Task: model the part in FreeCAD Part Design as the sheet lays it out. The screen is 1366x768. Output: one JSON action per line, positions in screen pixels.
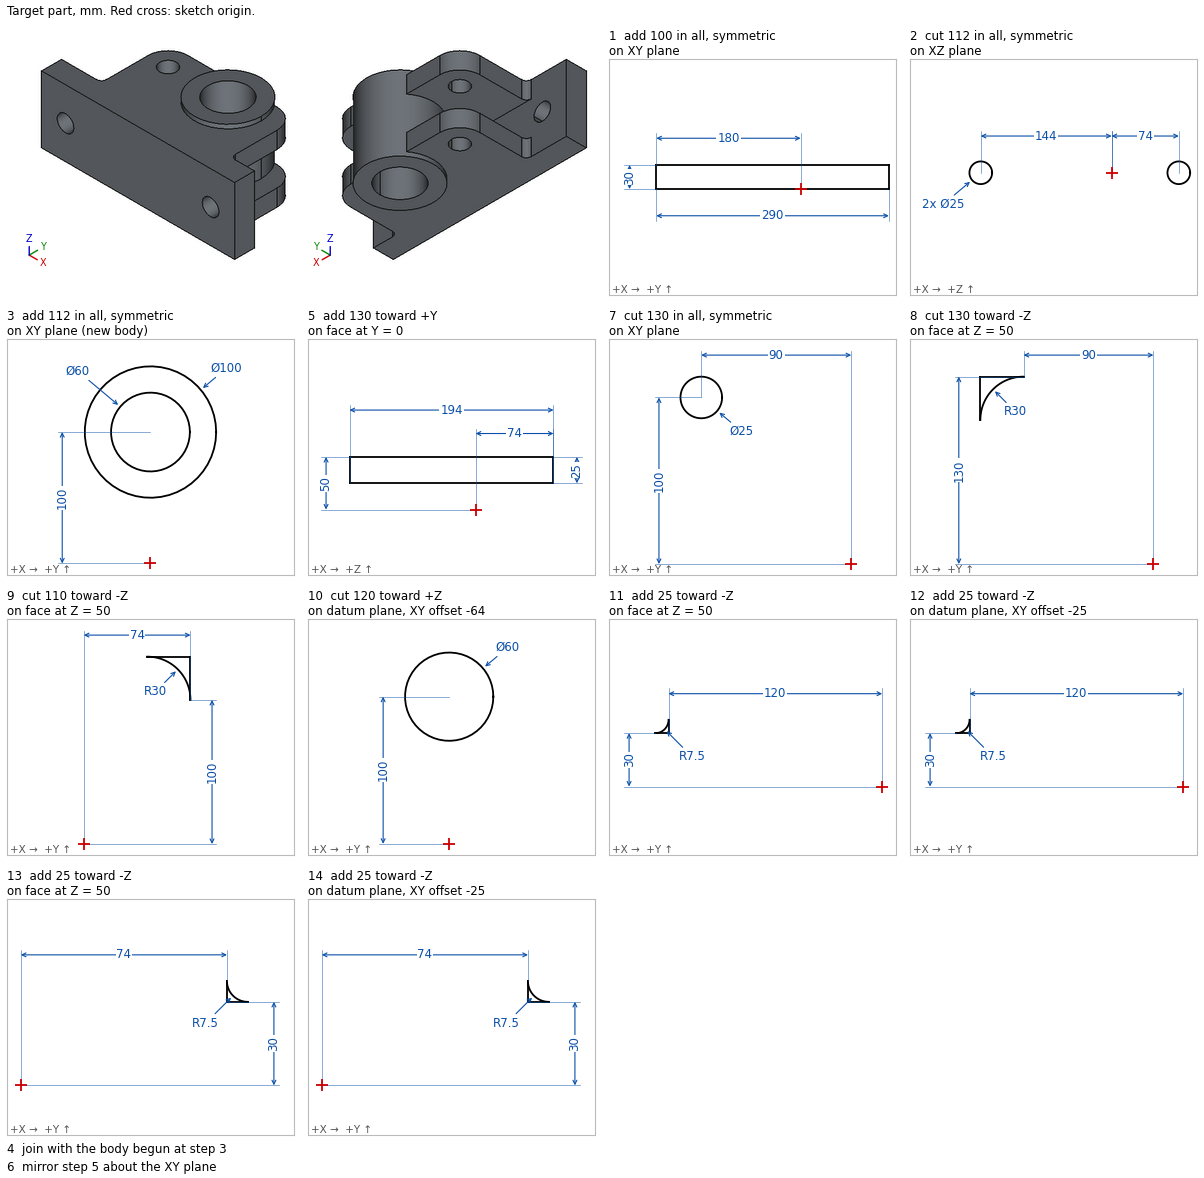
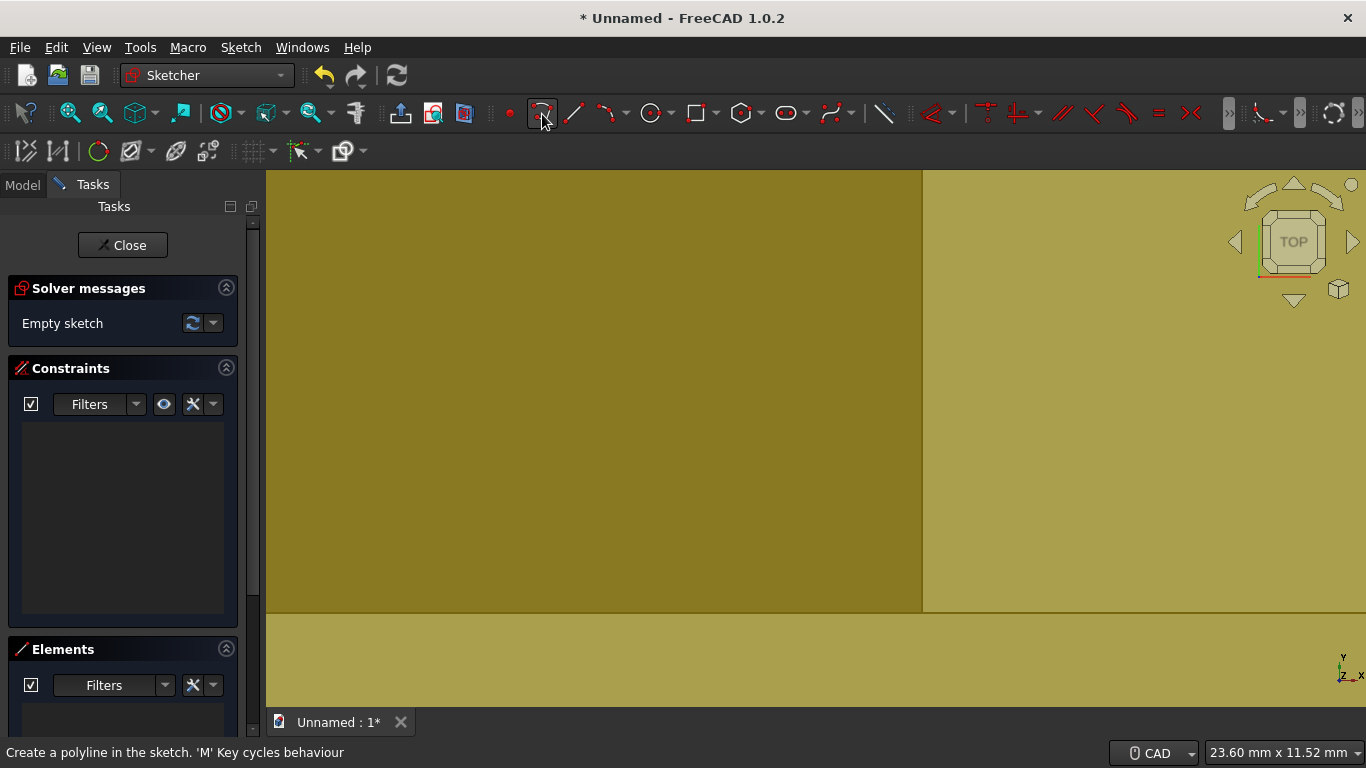
{"action": "left_click", "coordinate": [572, 613]}
{"action": "left_click", "coordinate": [922, 613]}
{"action": "left_click", "coordinate": [922, 264]}
{"action": "right_click", "coordinate": [922, 264]}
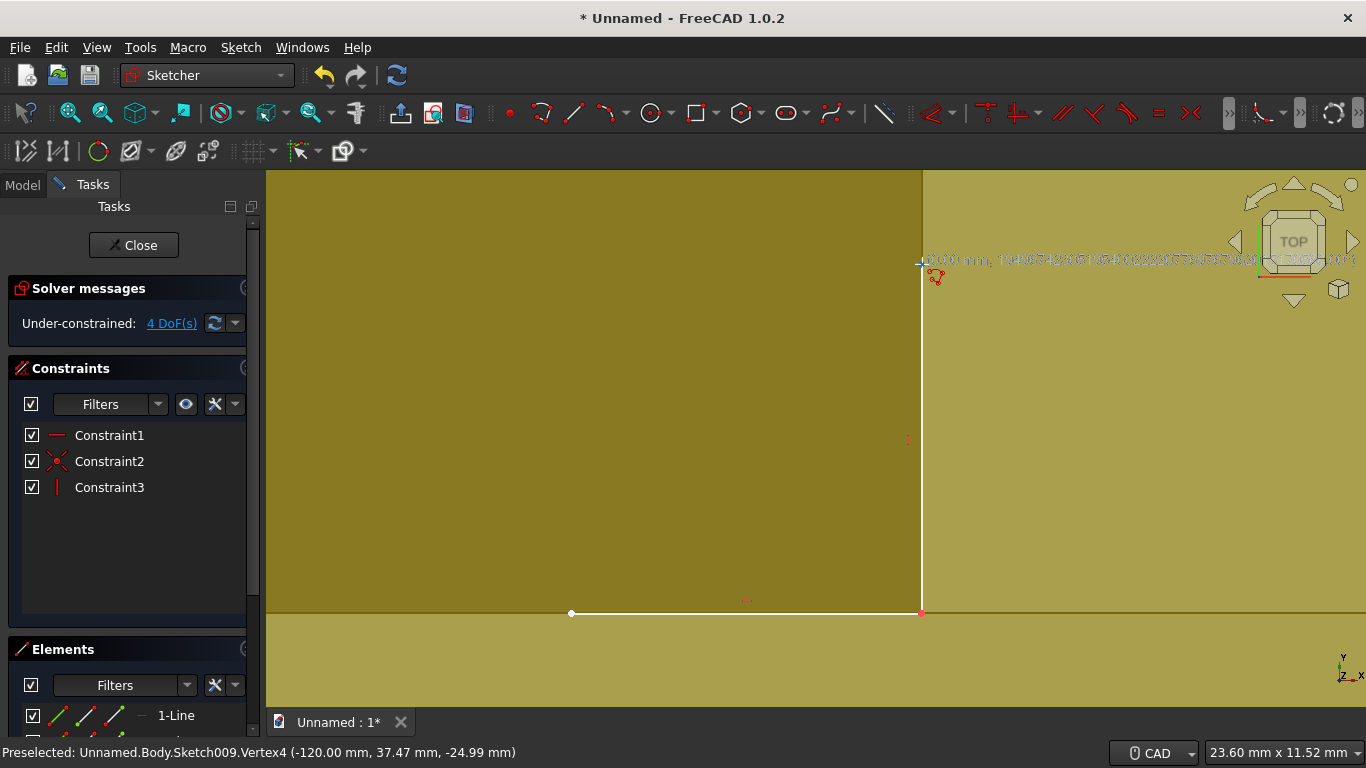
{"action": "left_click", "coordinate": [606, 114]}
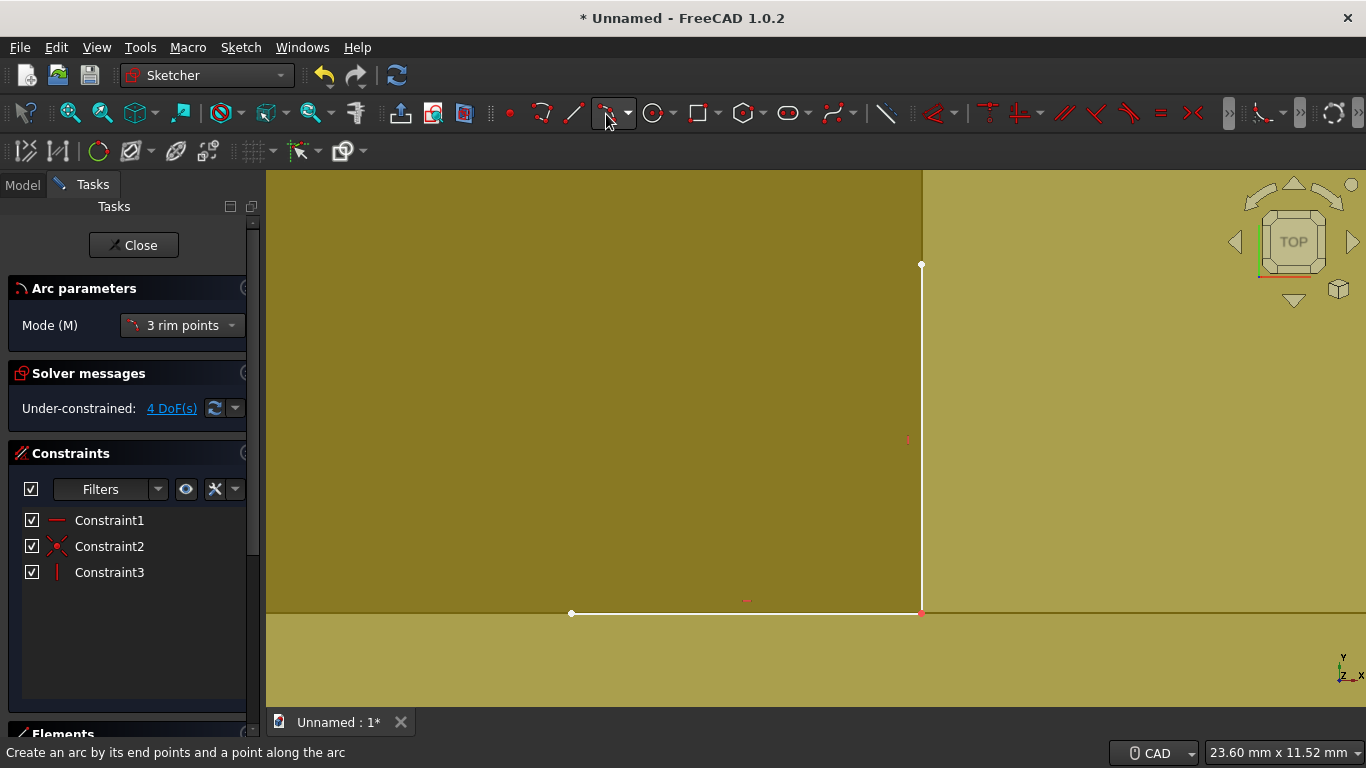
{"action": "left_click", "coordinate": [922, 265]}
{"action": "left_click", "coordinate": [572, 614]}
{"action": "left_click", "coordinate": [820, 511]}
{"action": "key", "text": "Escape"}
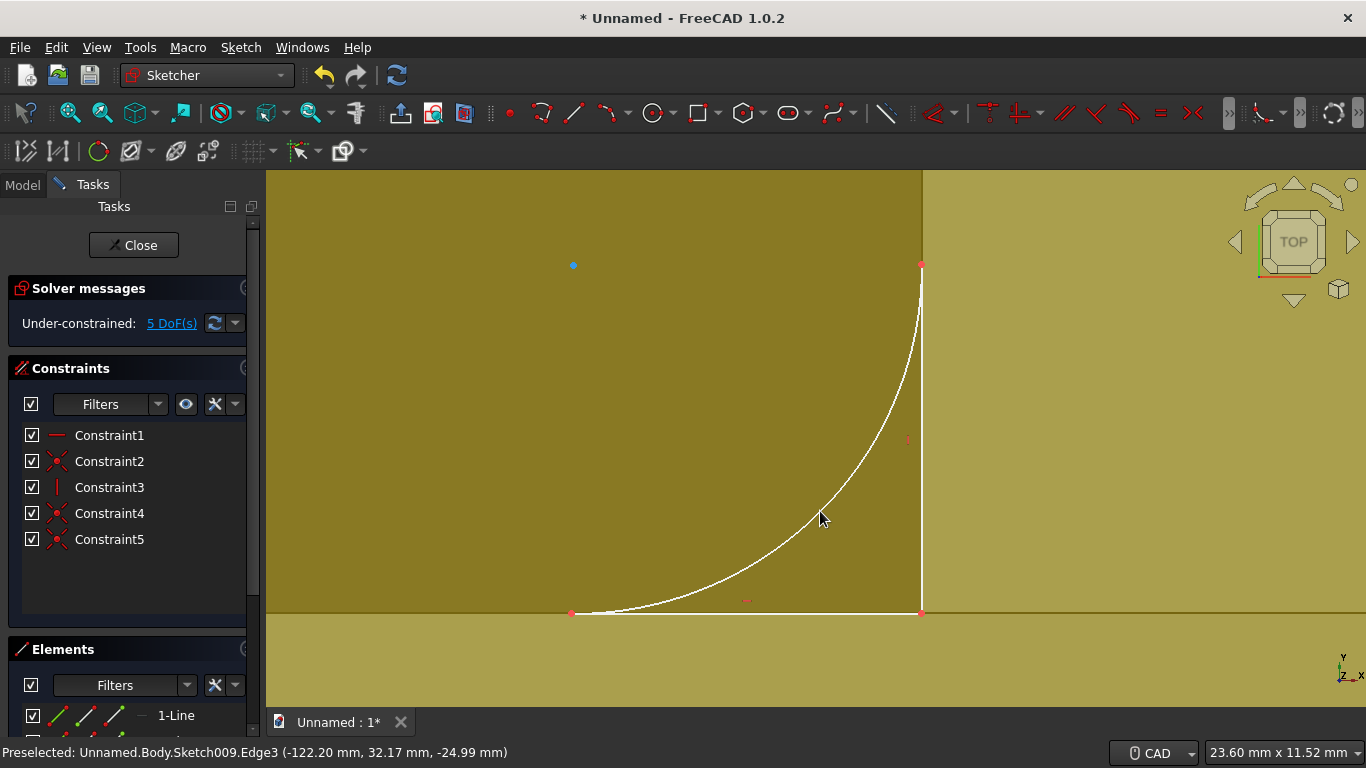
{"action": "left_click", "coordinate": [677, 614]}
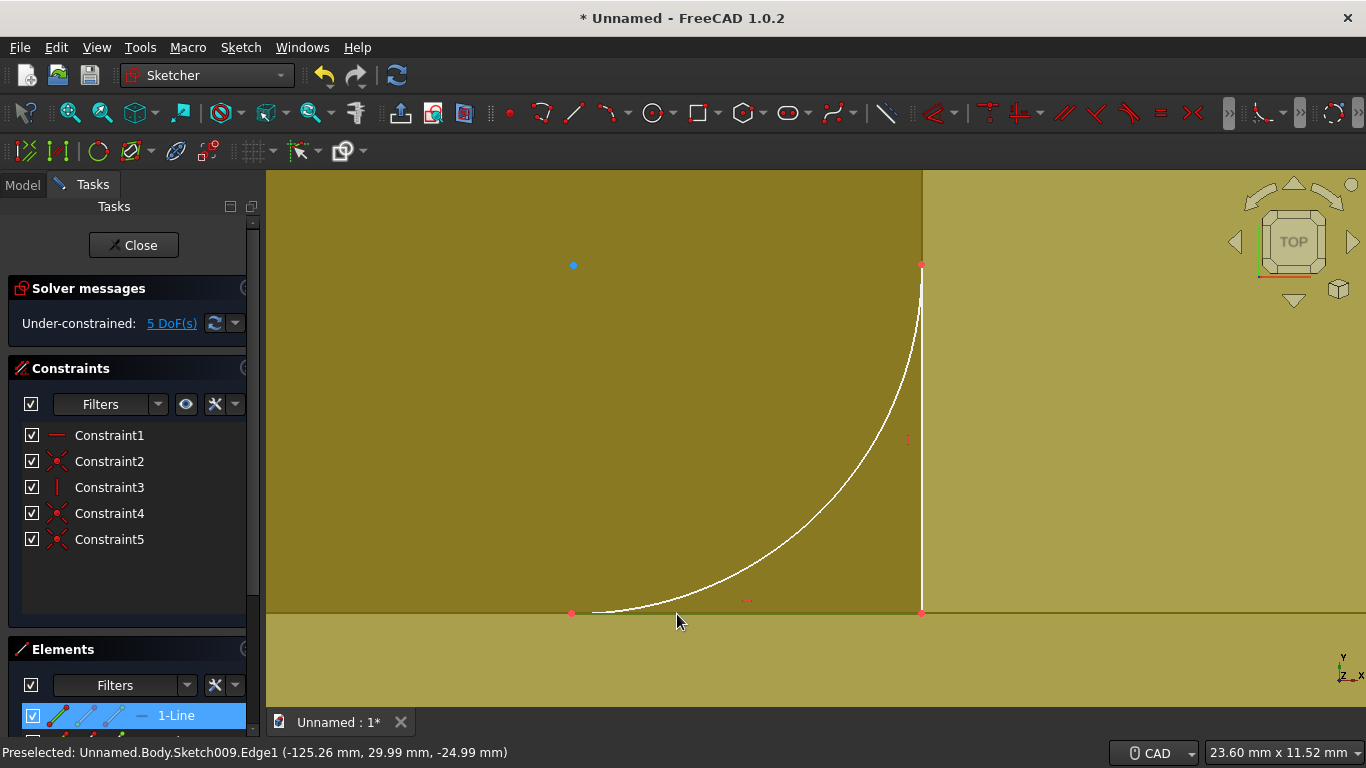
{"action": "left_click", "coordinate": [731, 576]}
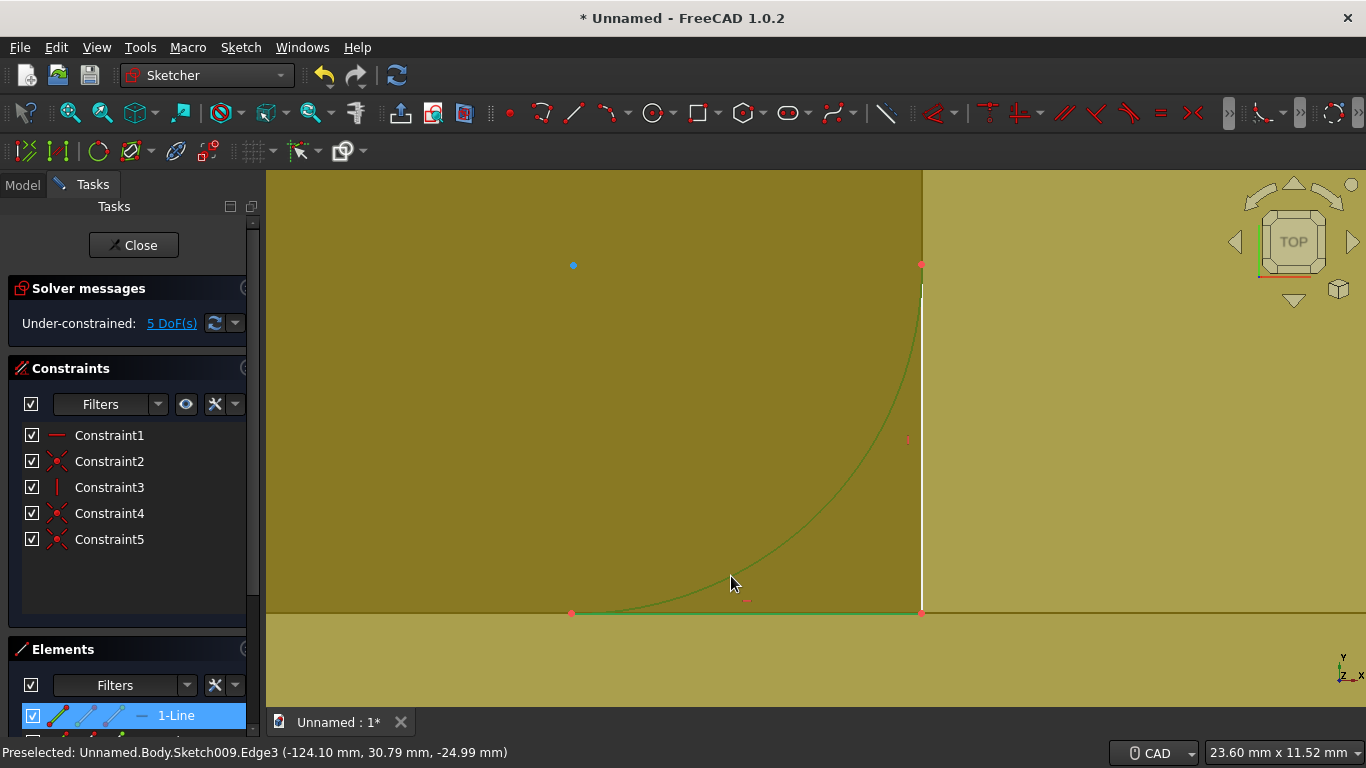
{"action": "left_click", "coordinate": [1130, 114]}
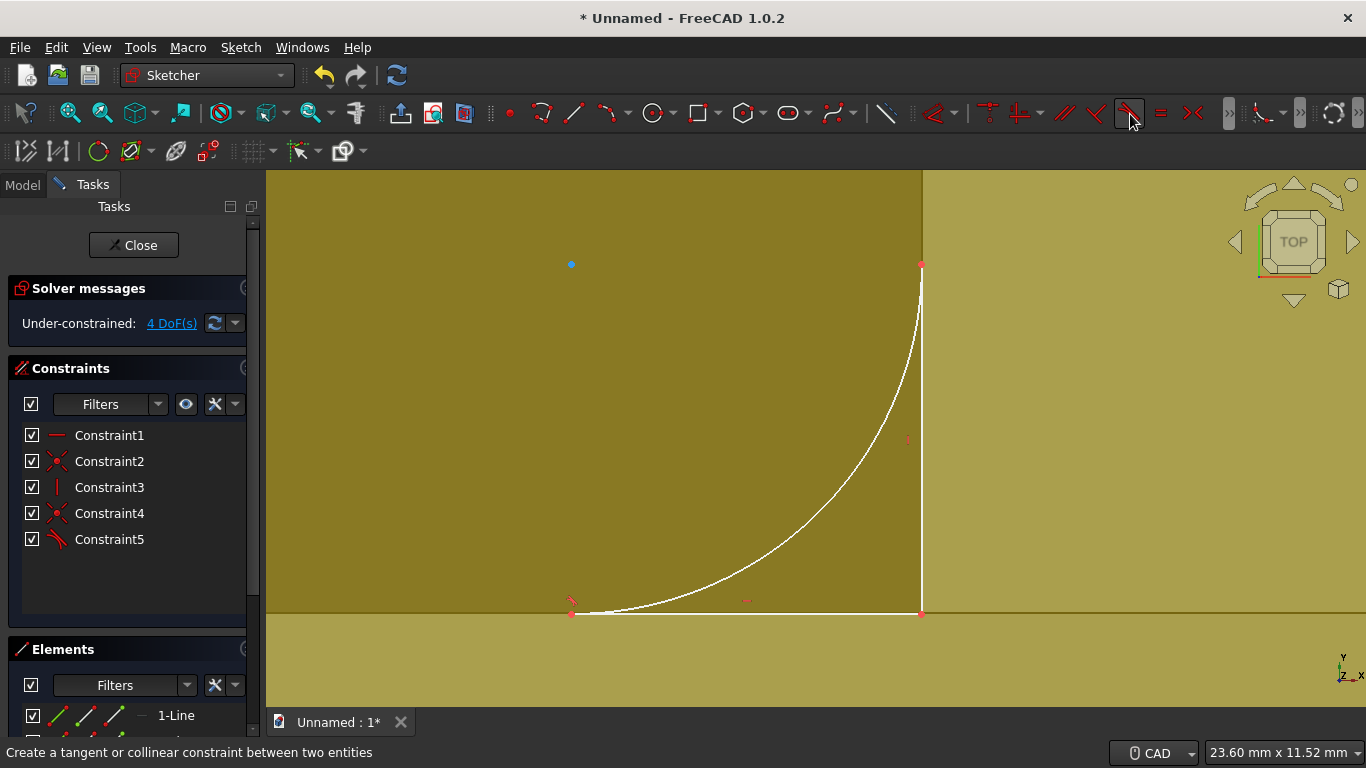
{"action": "left_click", "coordinate": [922, 509]}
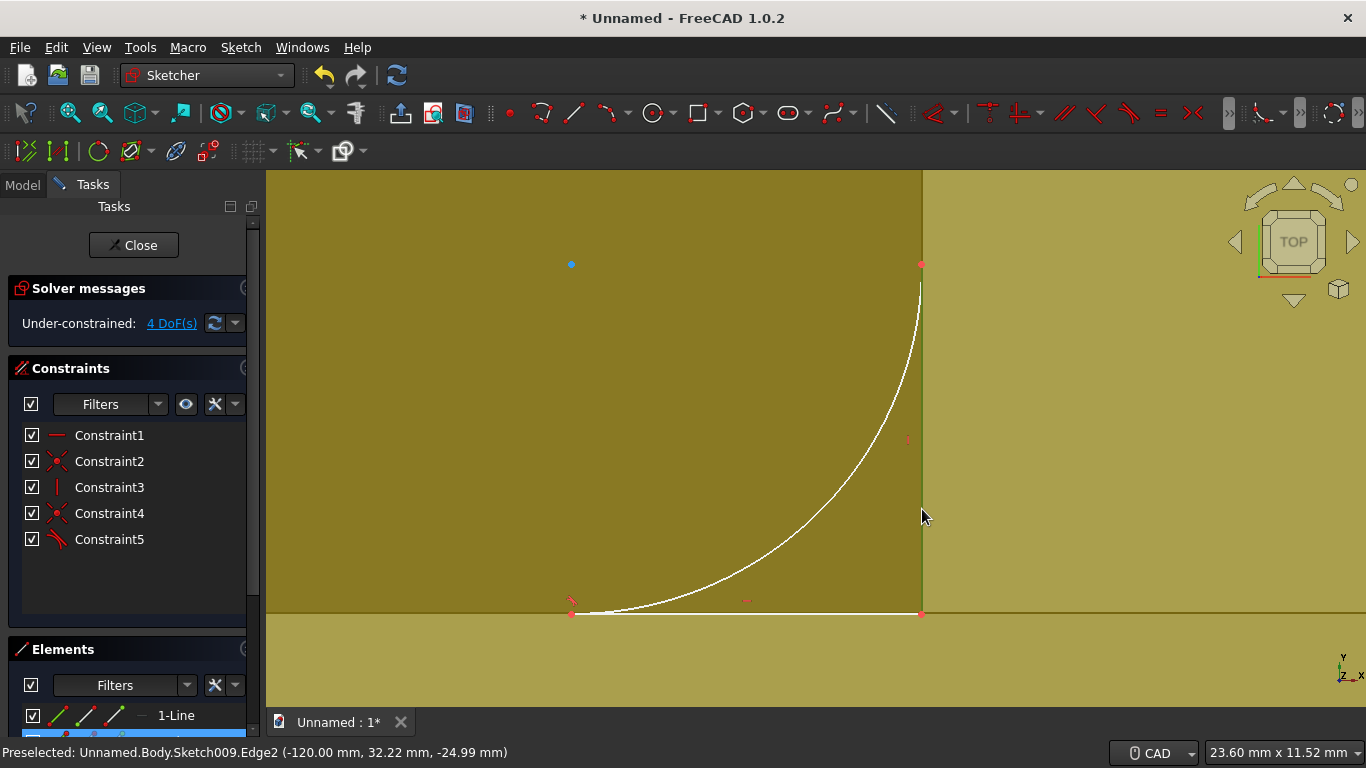
{"action": "left_click", "coordinate": [731, 576]}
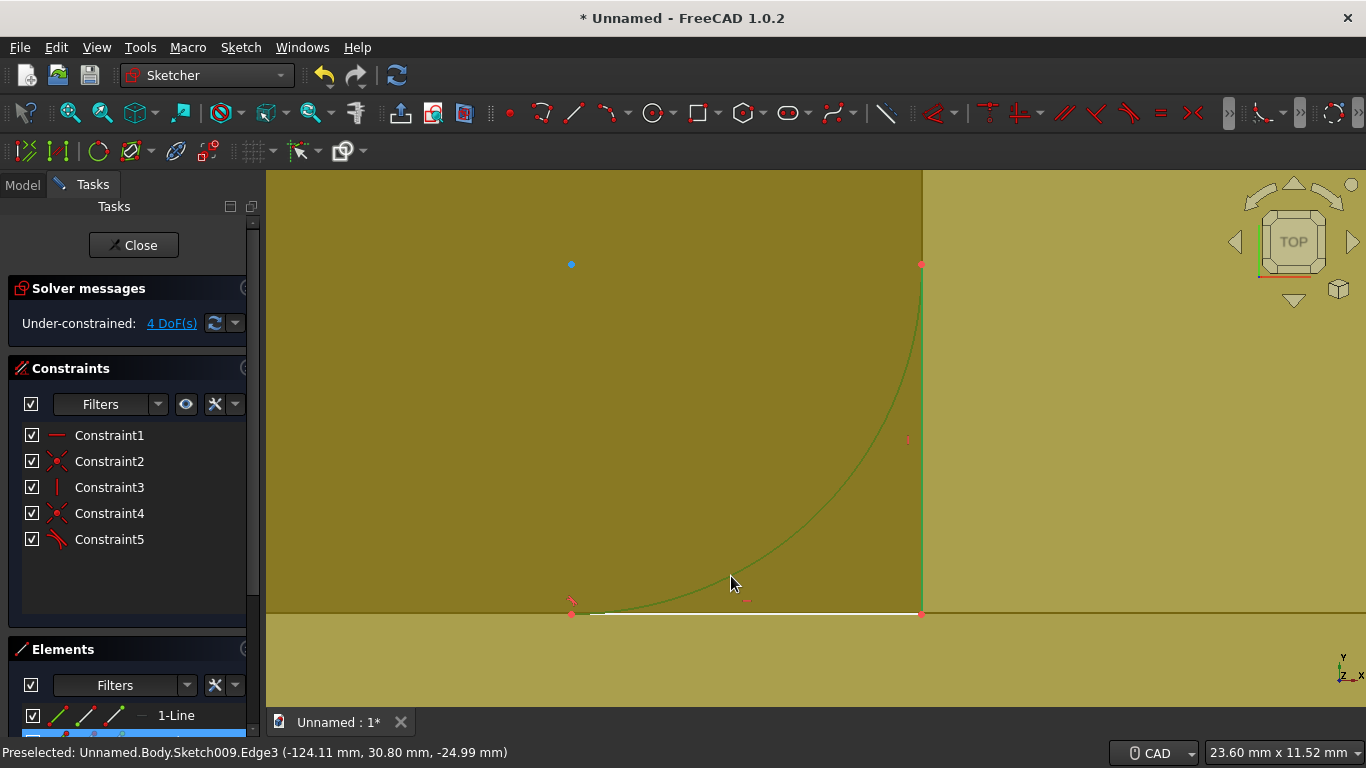
{"action": "left_click", "coordinate": [1130, 114]}